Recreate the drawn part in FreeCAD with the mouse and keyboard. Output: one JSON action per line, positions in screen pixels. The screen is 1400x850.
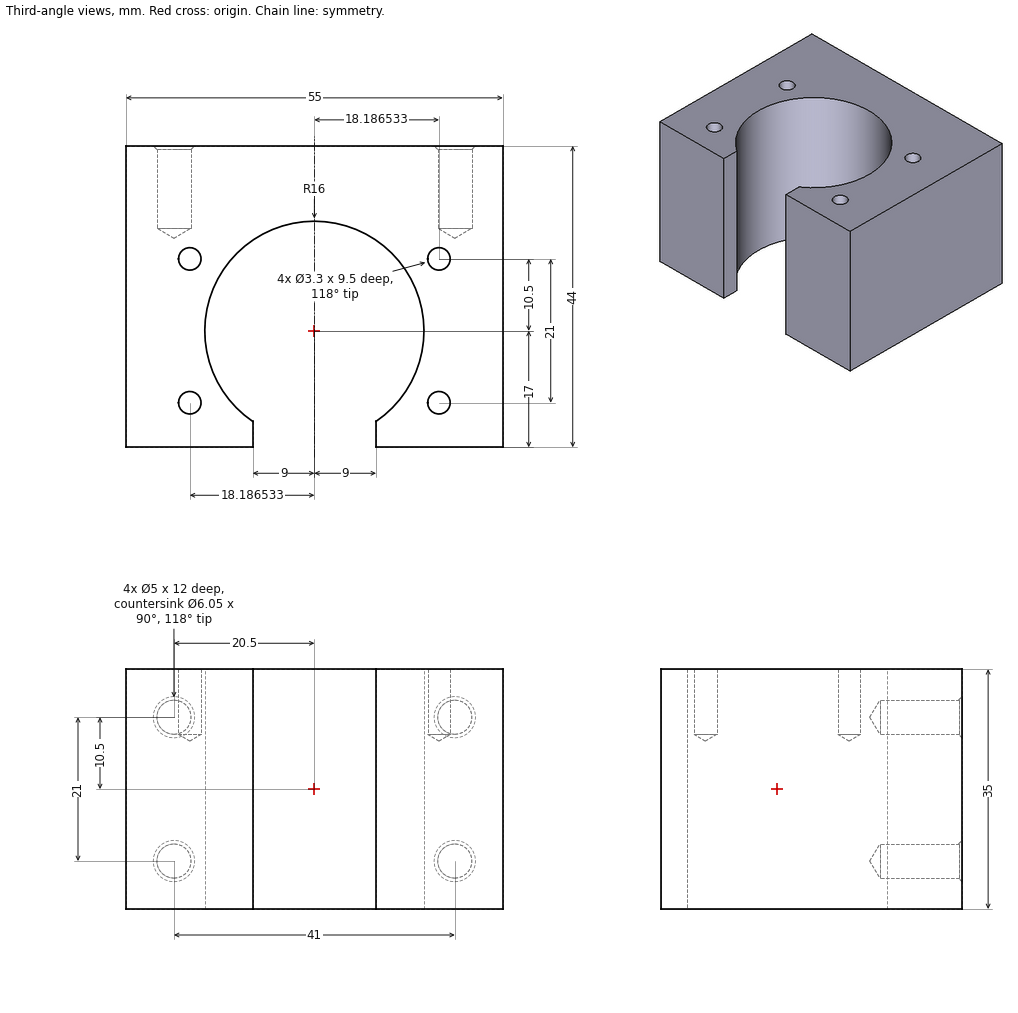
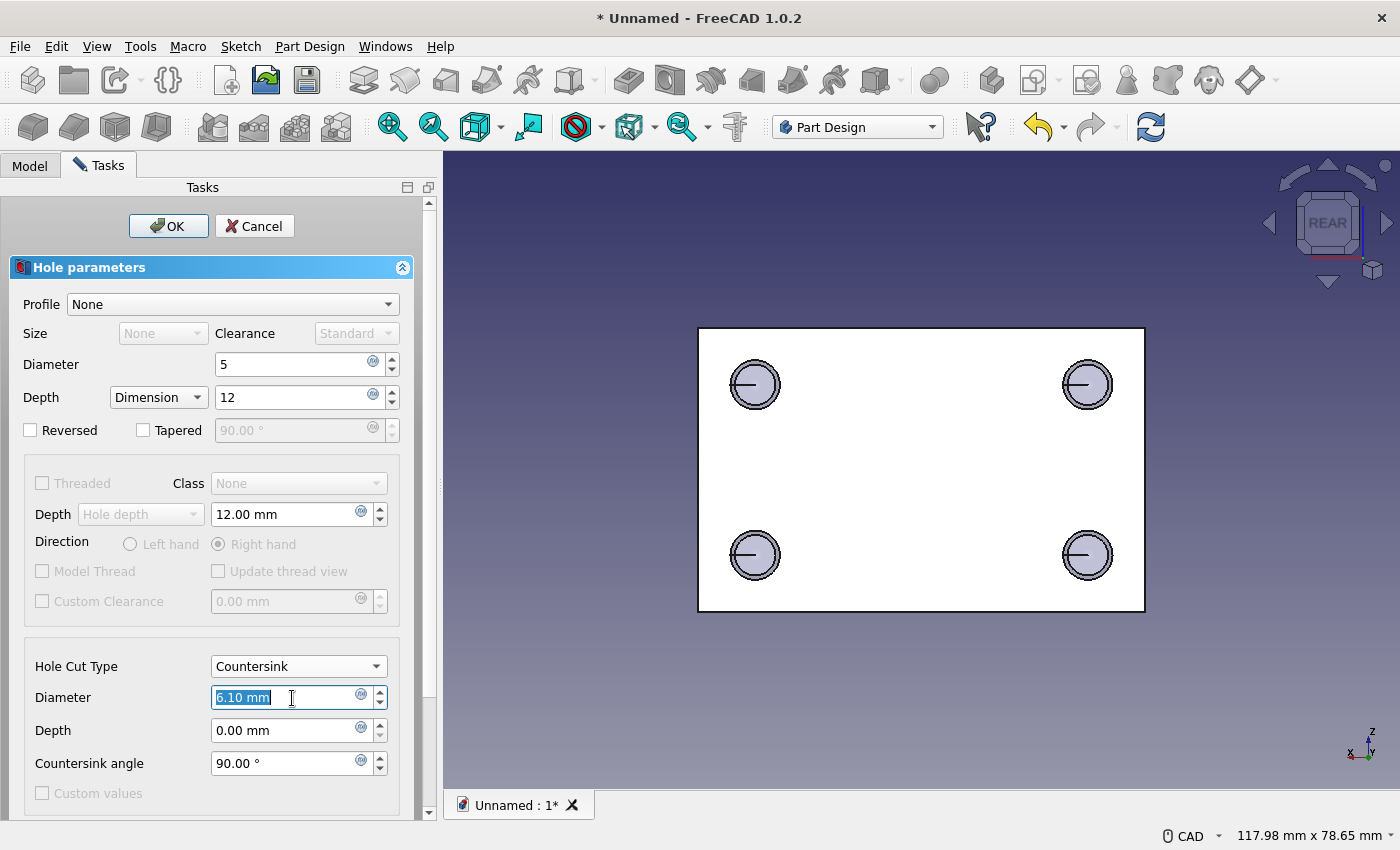
{"action": "type", "text": "6.05"}
{"action": "key", "text": "Tab"}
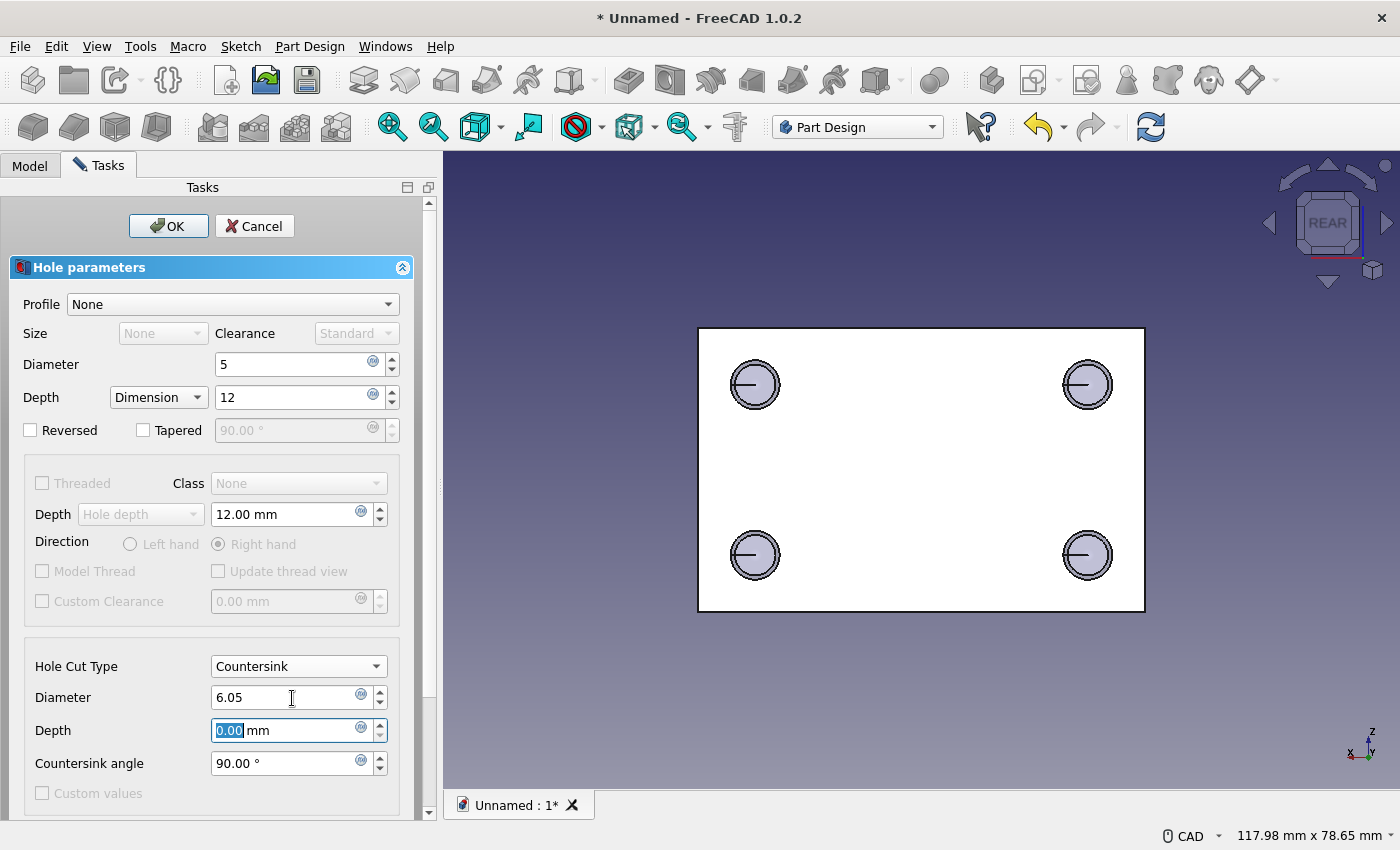
{"action": "left_click", "coordinate": [169, 226]}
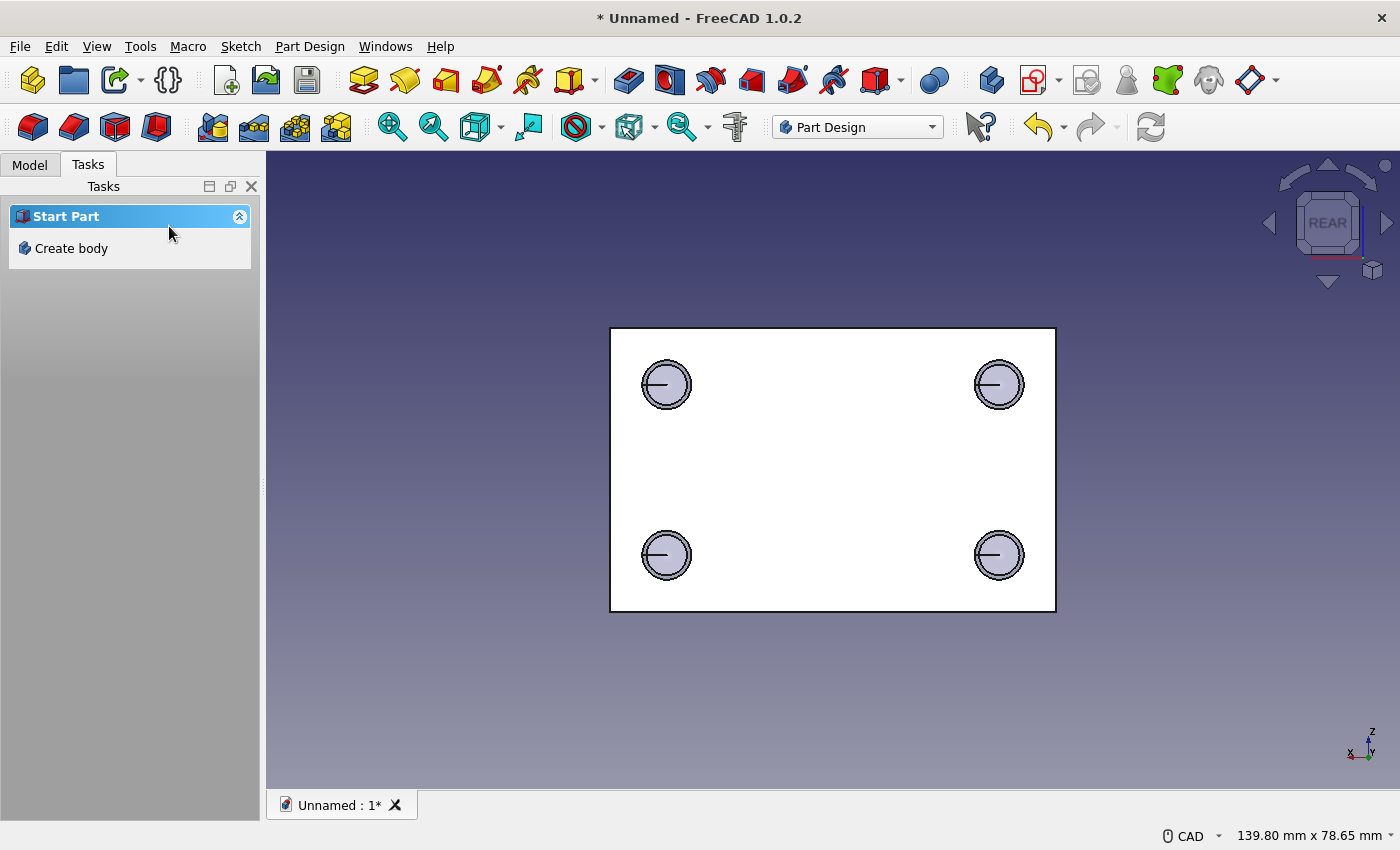
{"action": "key", "text": "0"}